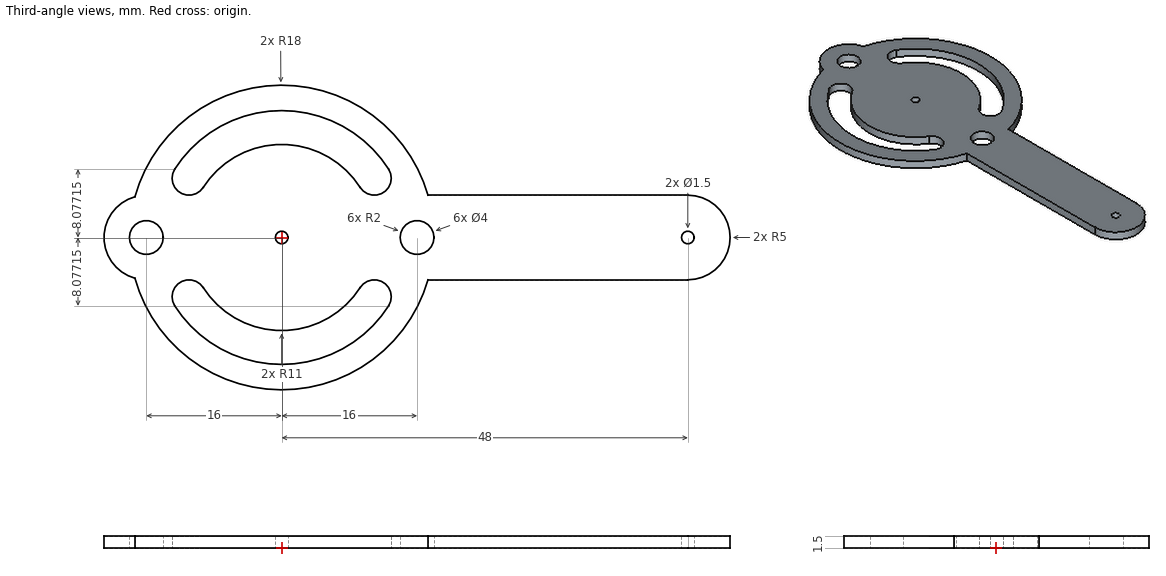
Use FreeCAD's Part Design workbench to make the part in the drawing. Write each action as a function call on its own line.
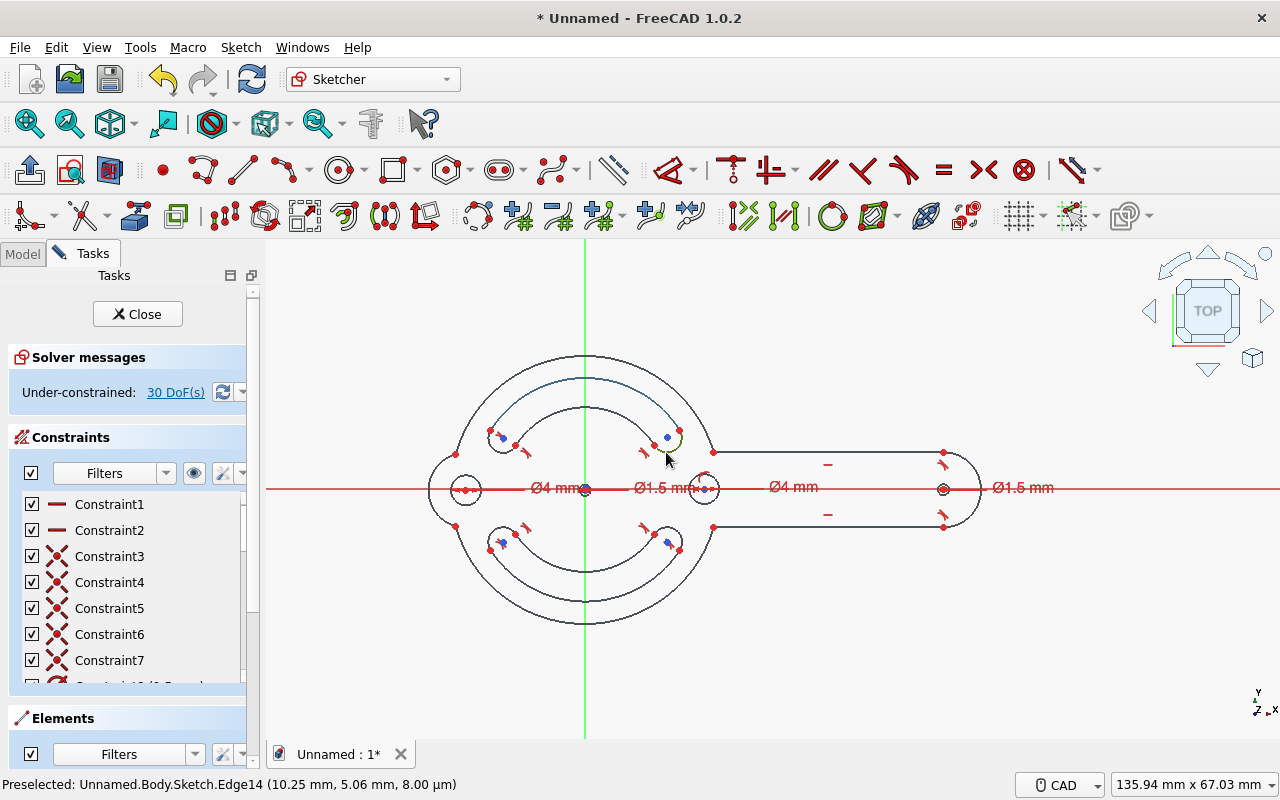
click(904, 170)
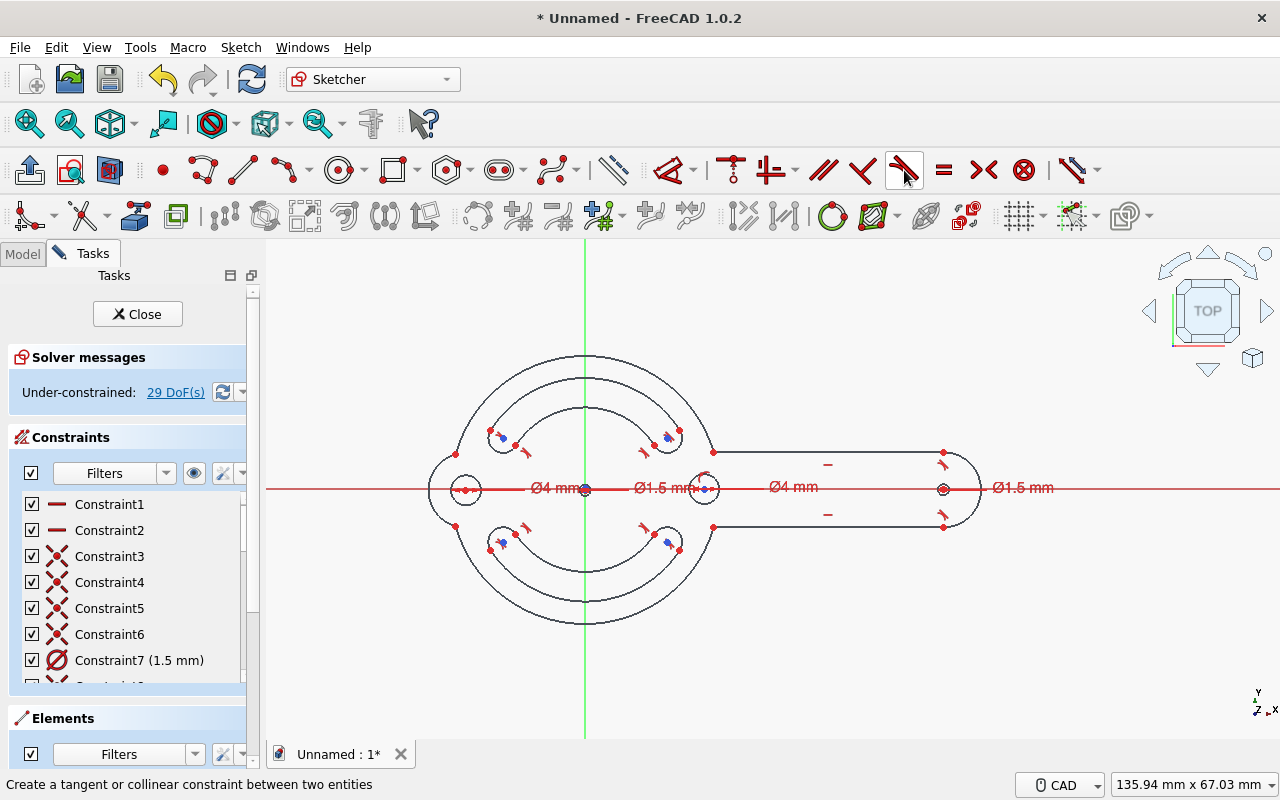
scroll(589, 486, up, 5)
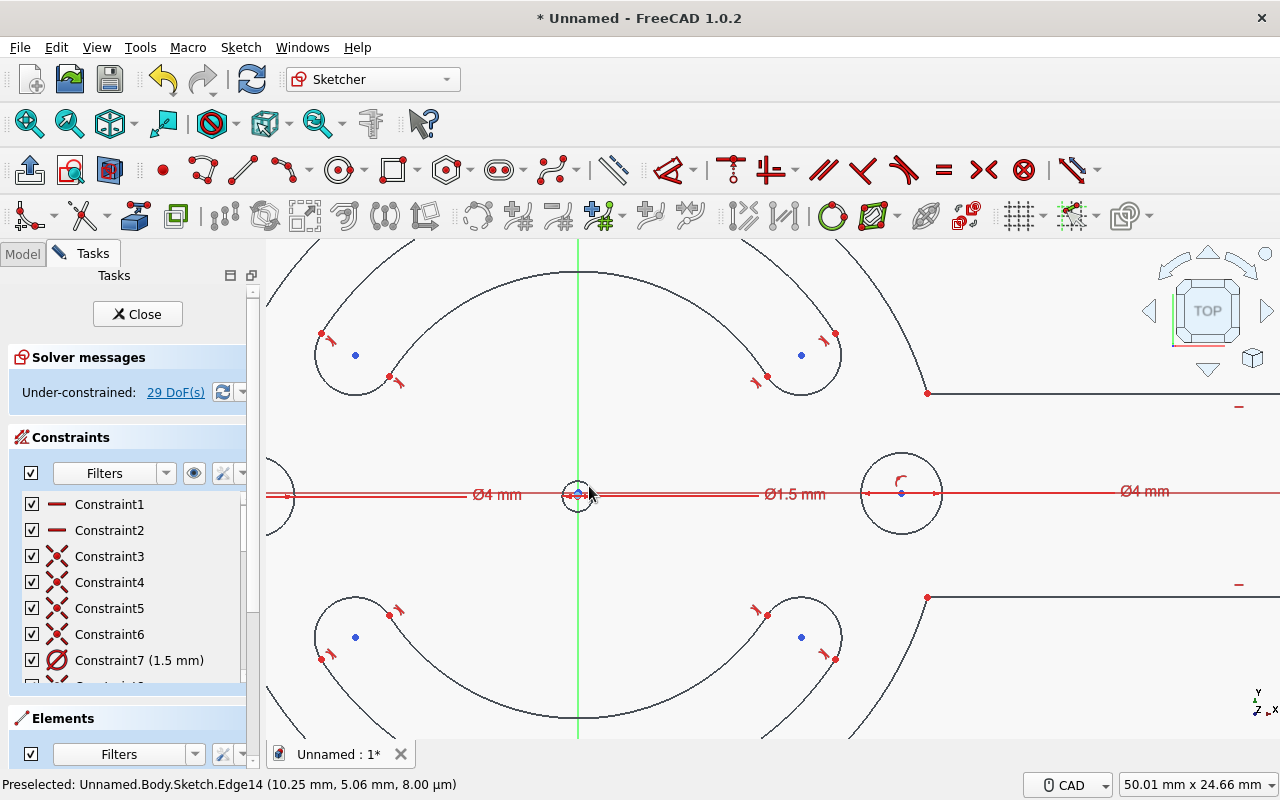
click(588, 486)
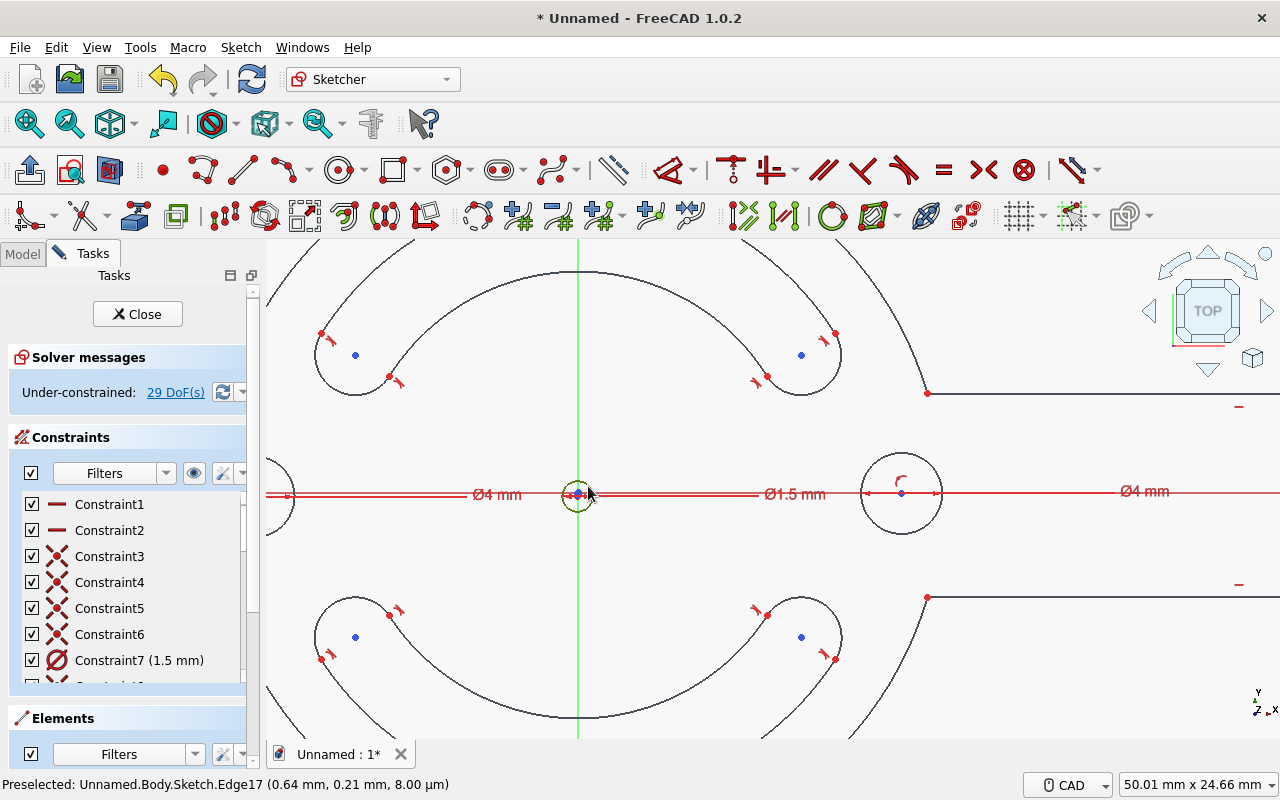
scroll(589, 486, down, 5)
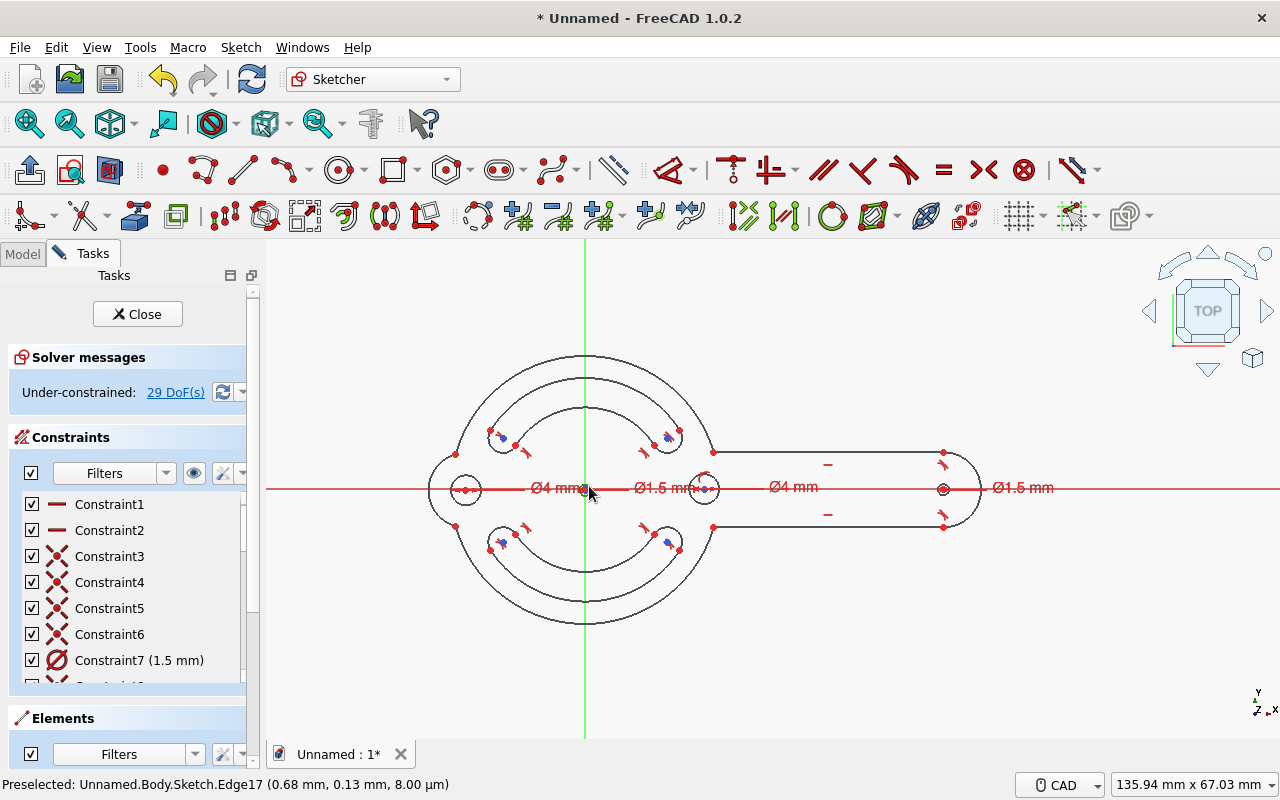
click(518, 606)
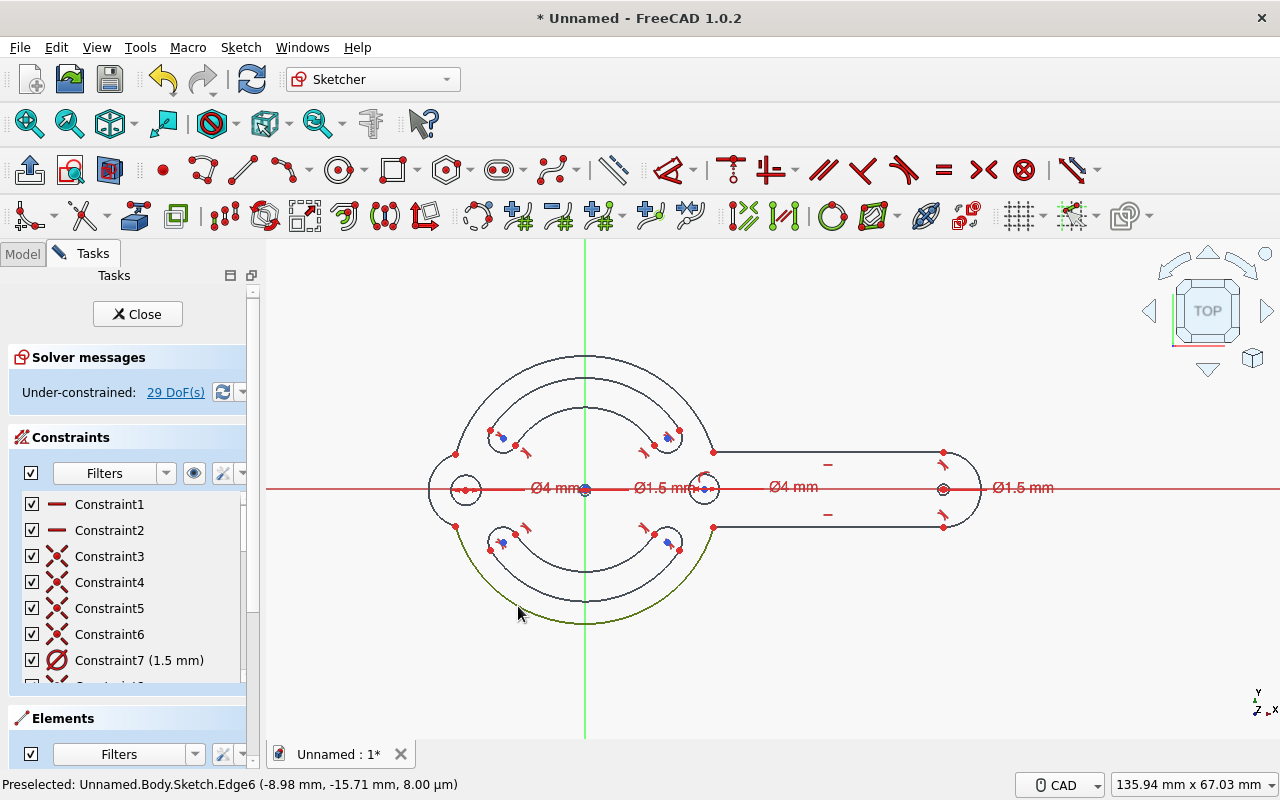
click(732, 170)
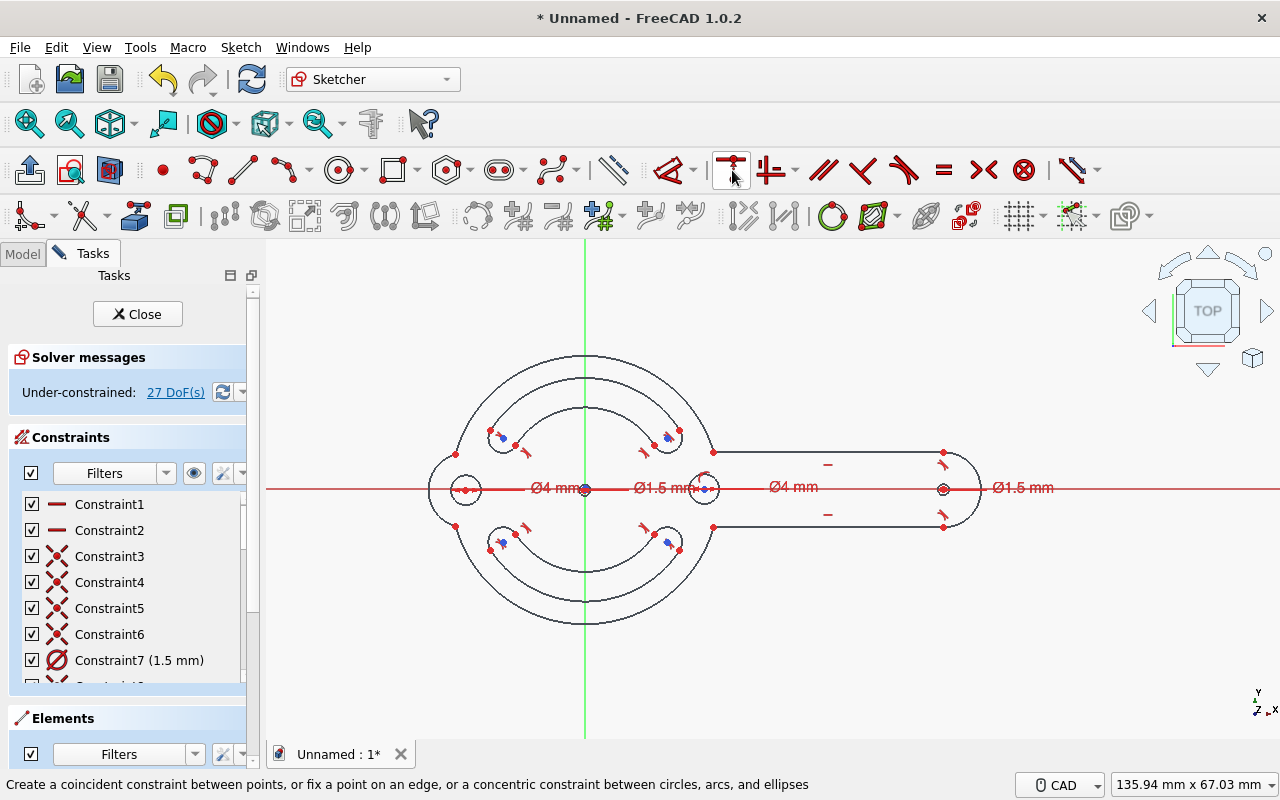
scroll(589, 486, up, 5)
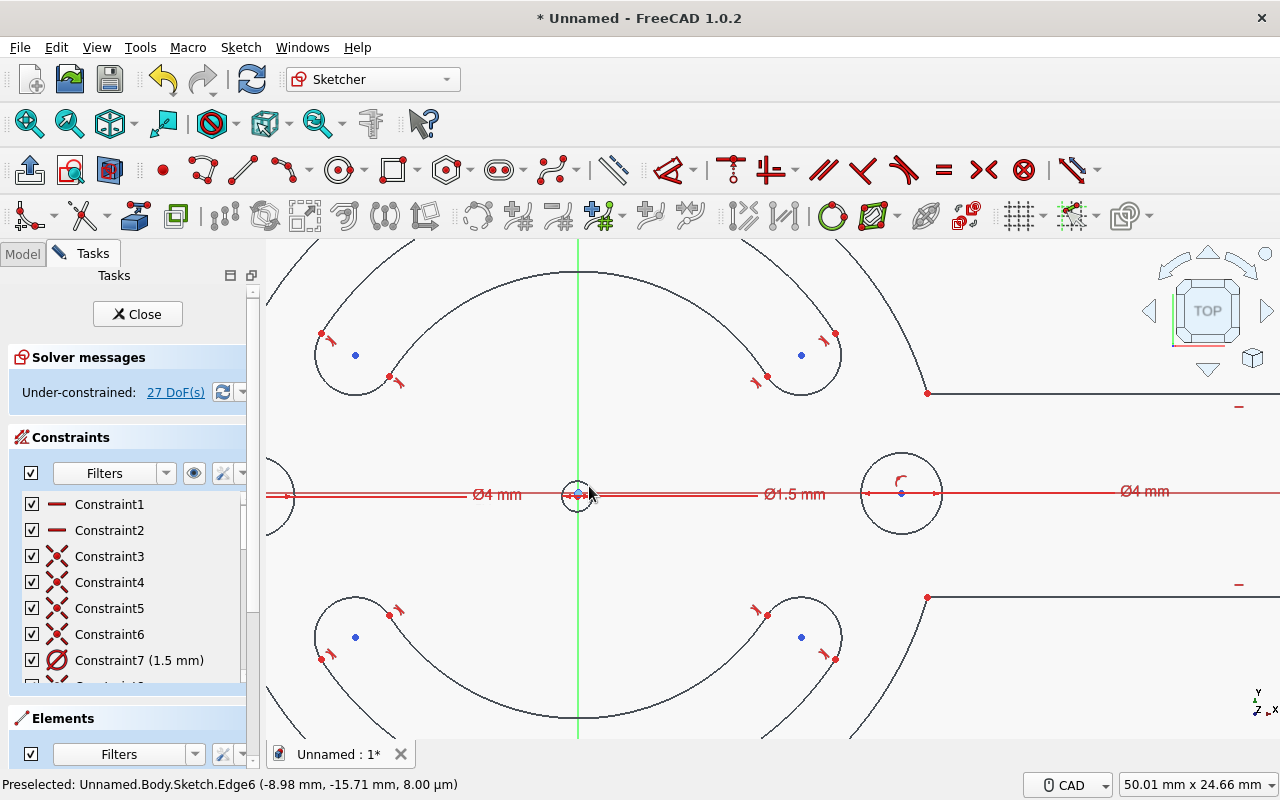
click(588, 486)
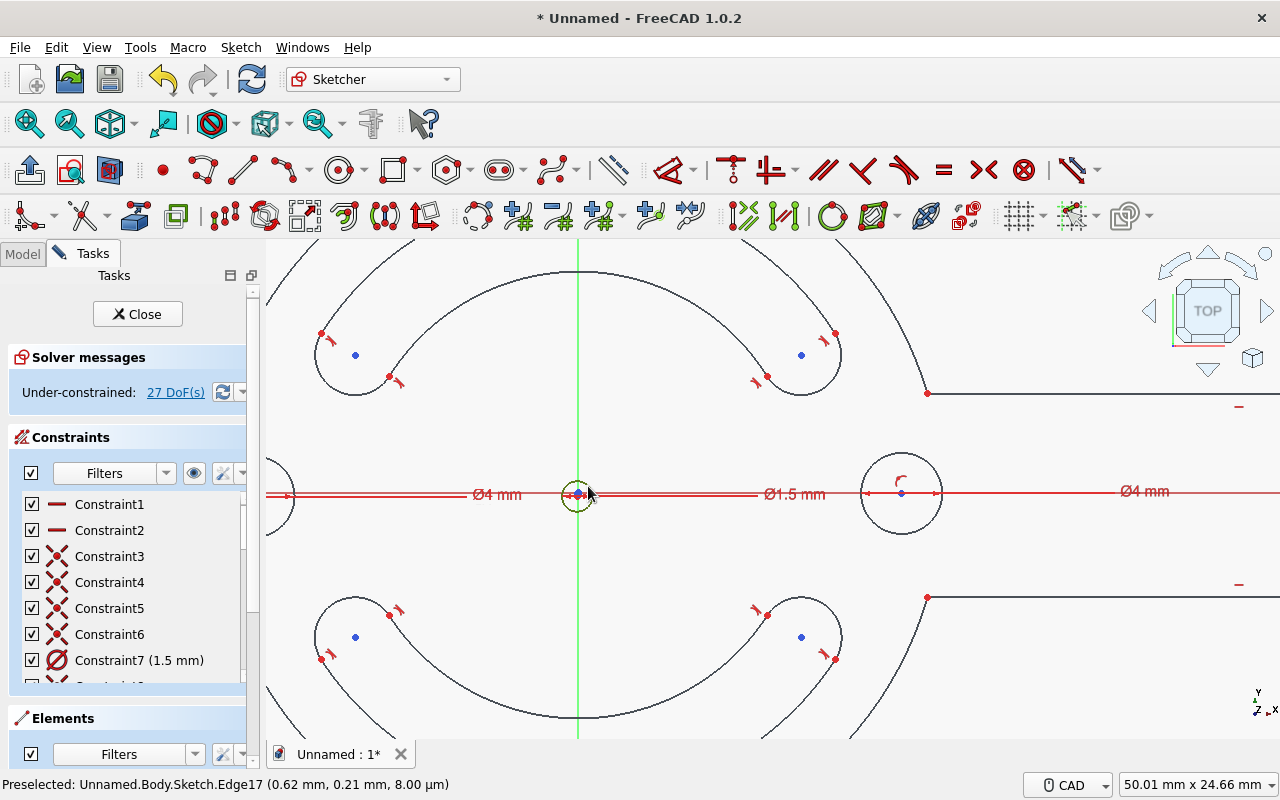
click(491, 701)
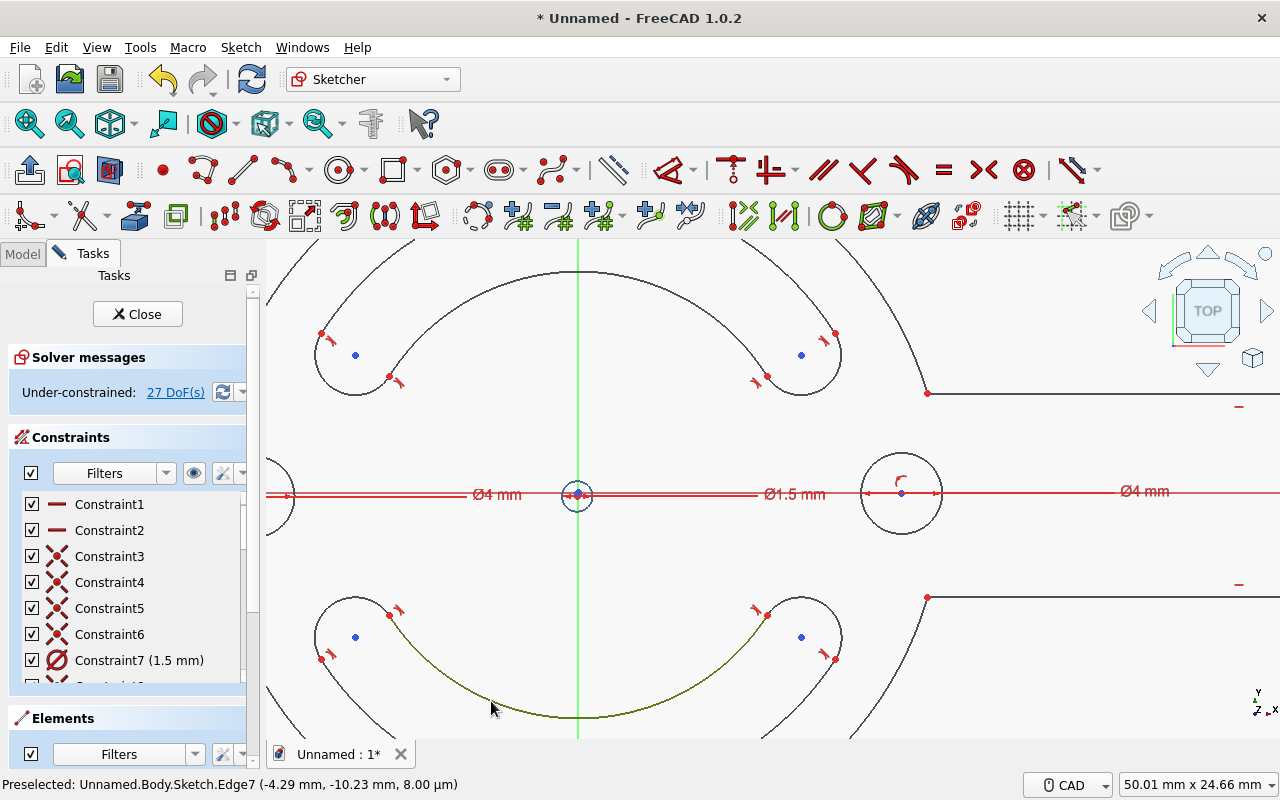
click(732, 170)